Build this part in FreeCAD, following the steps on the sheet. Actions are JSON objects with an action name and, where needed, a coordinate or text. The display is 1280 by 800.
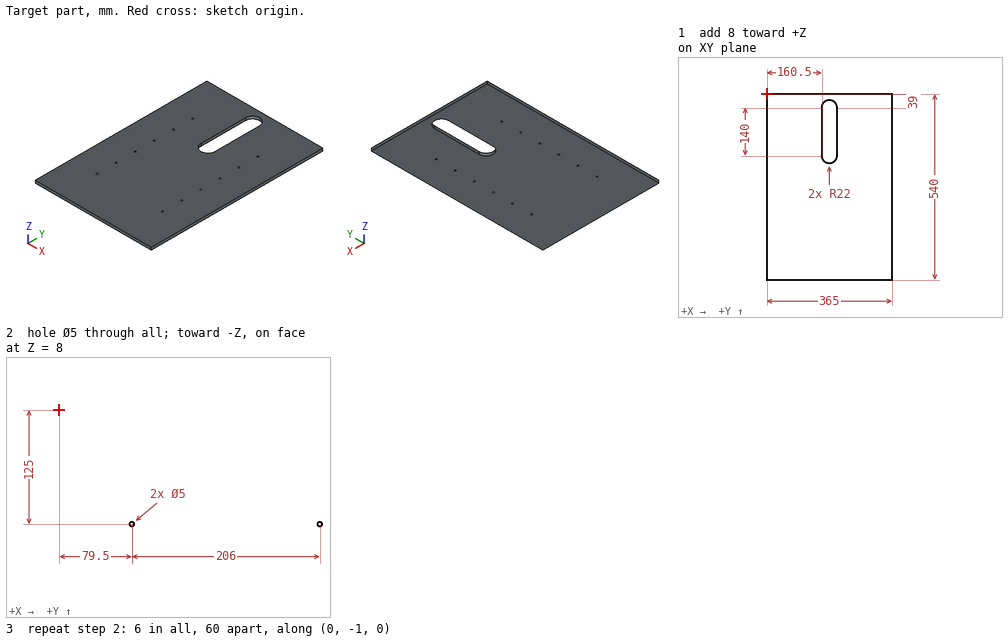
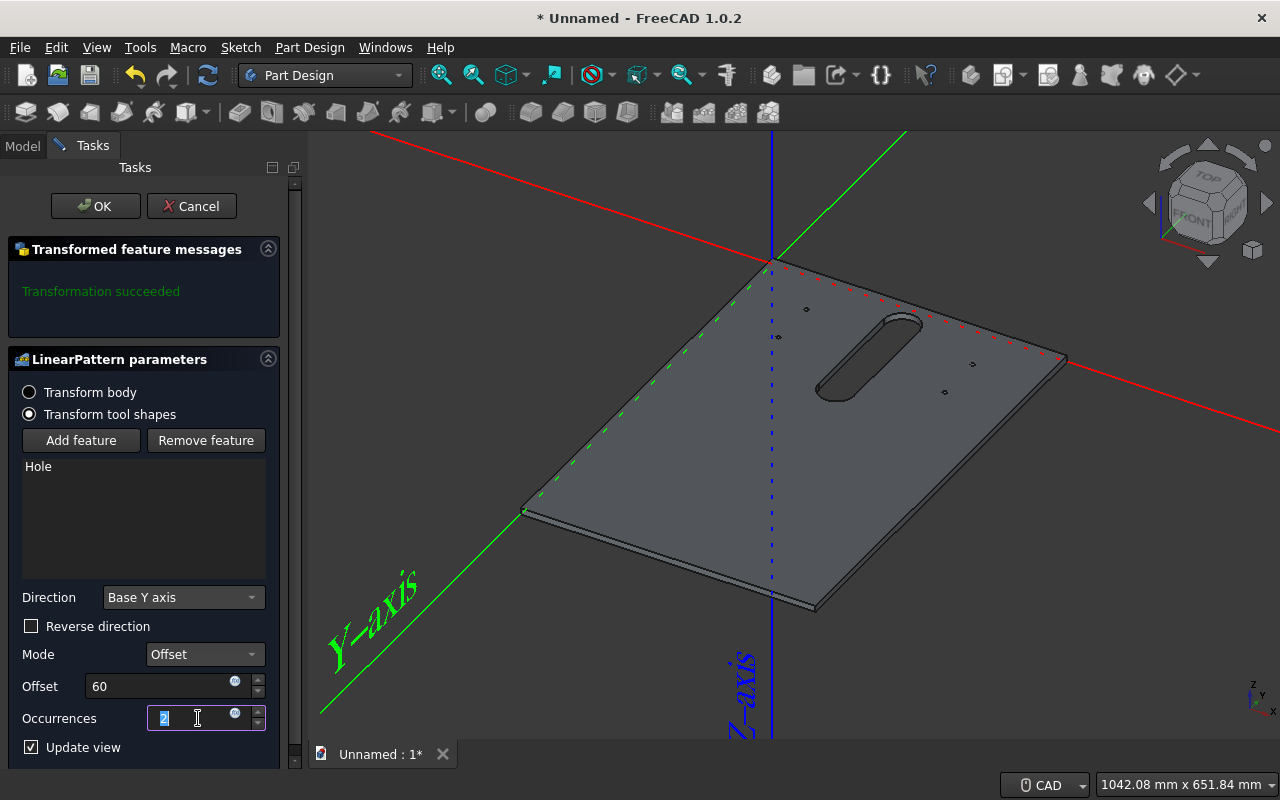
{"action": "type", "text": "6"}
{"action": "key", "text": "Tab"}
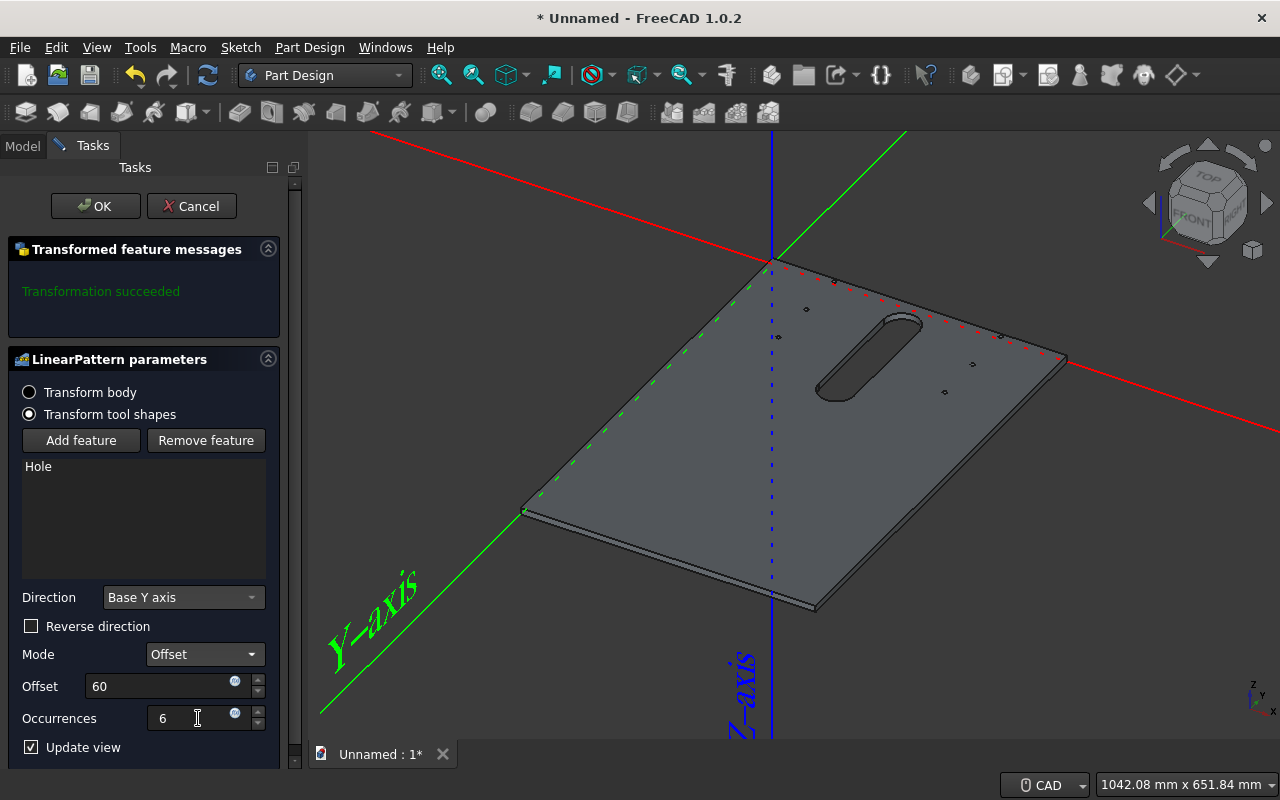
{"action": "left_click", "coordinate": [30, 626]}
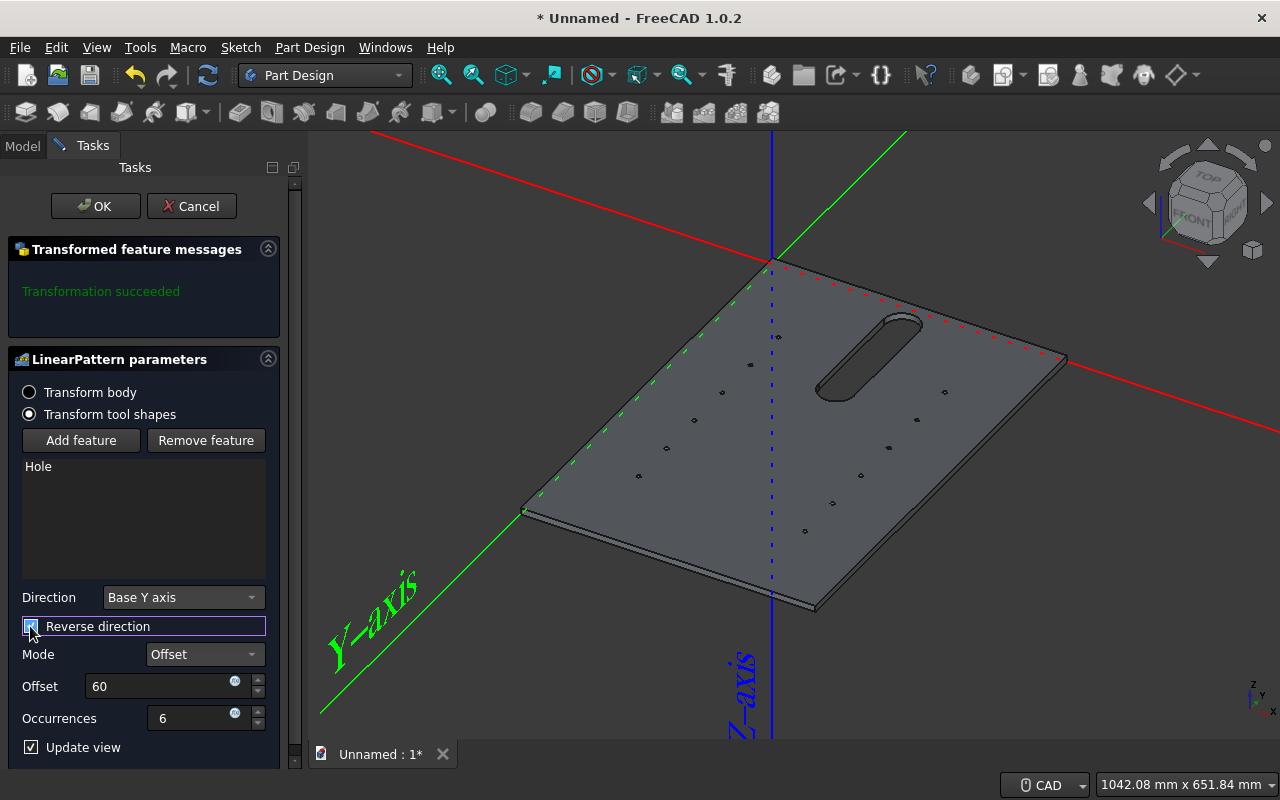
{"action": "left_click", "coordinate": [96, 206]}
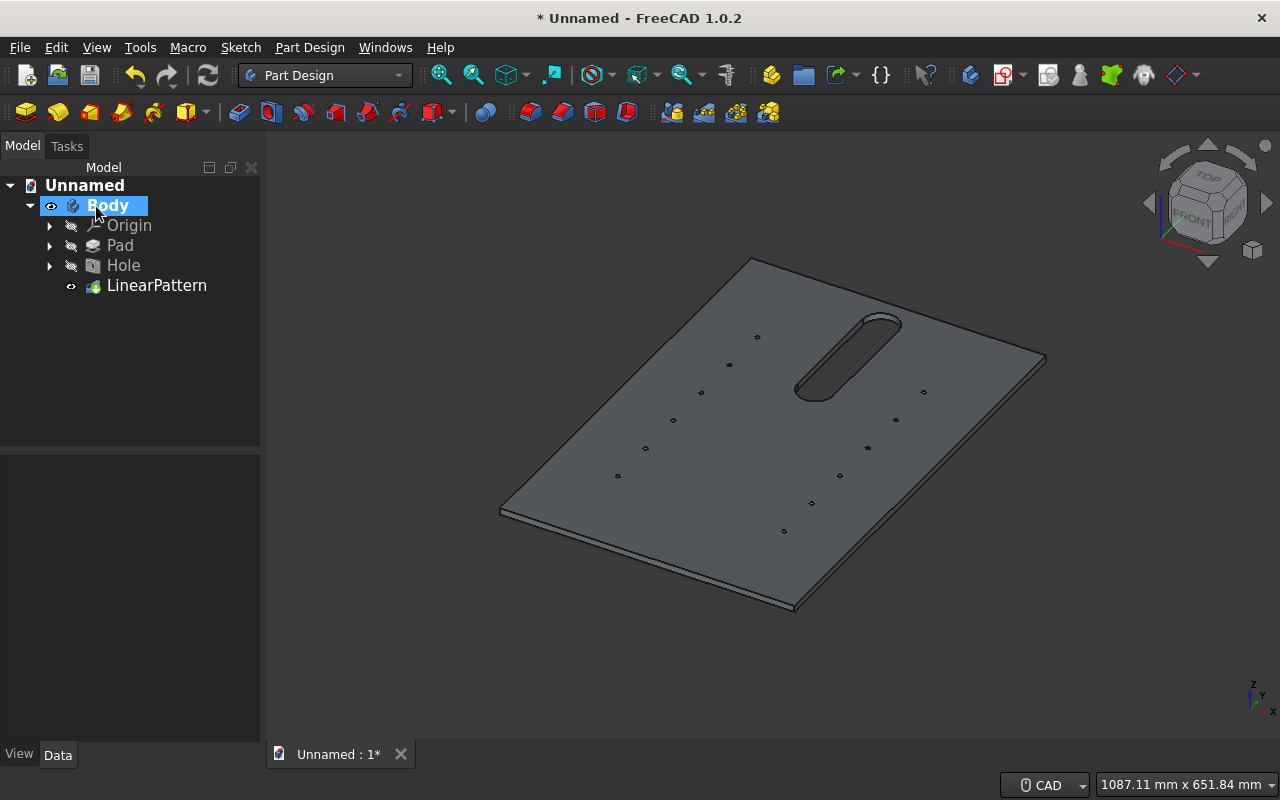
{"action": "key", "text": "0"}